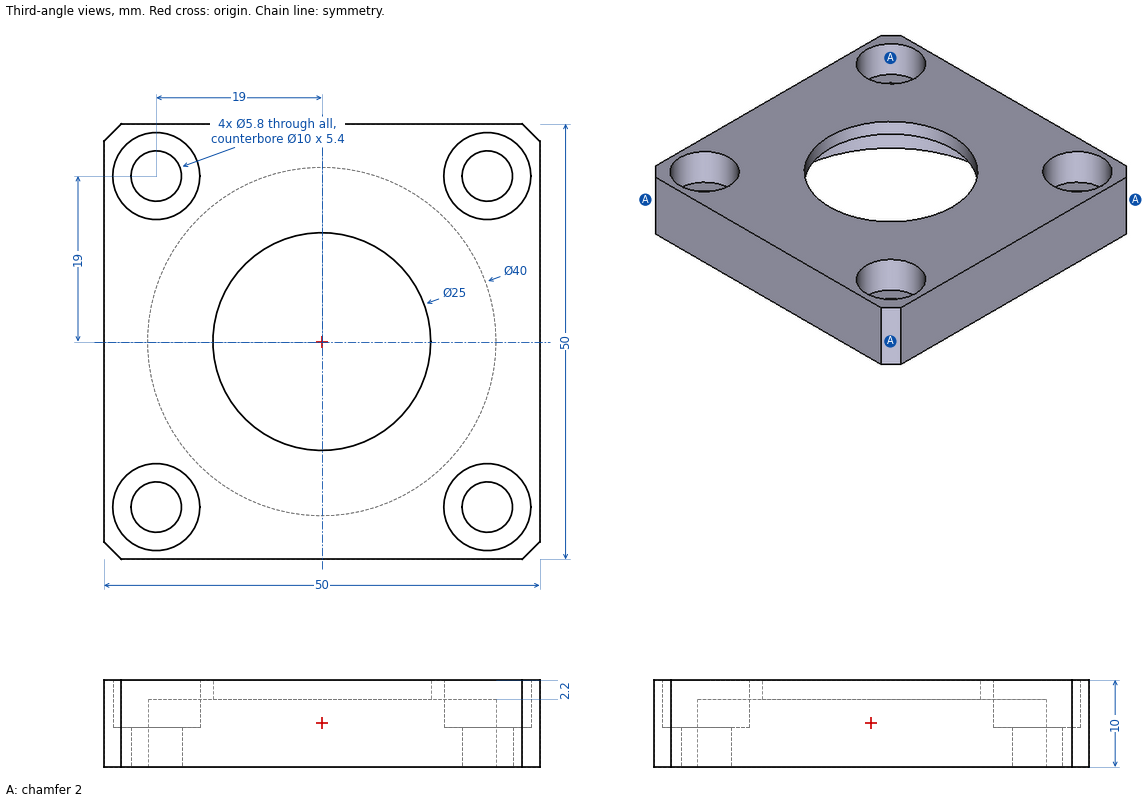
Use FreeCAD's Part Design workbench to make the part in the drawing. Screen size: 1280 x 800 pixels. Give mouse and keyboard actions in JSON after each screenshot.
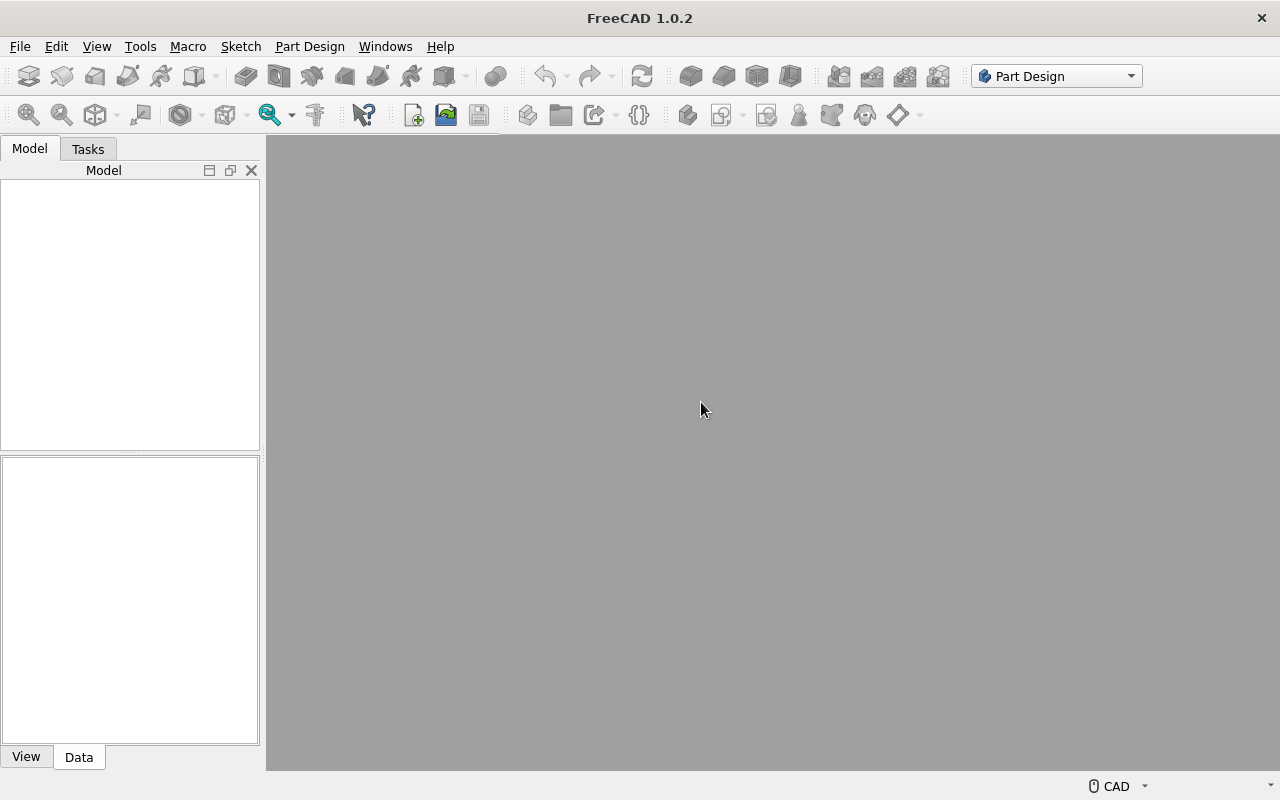
{"action": "left_click", "coordinate": [413, 116]}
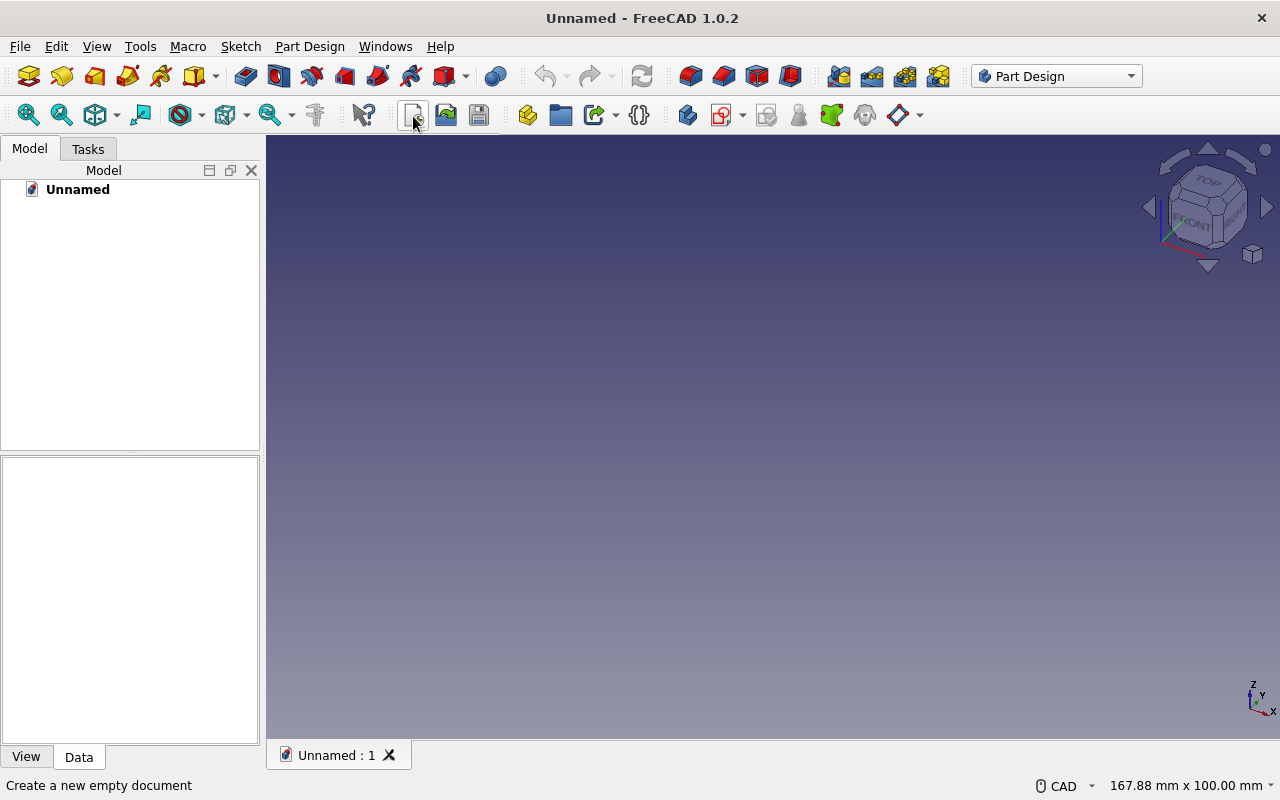
{"action": "left_click", "coordinate": [720, 116]}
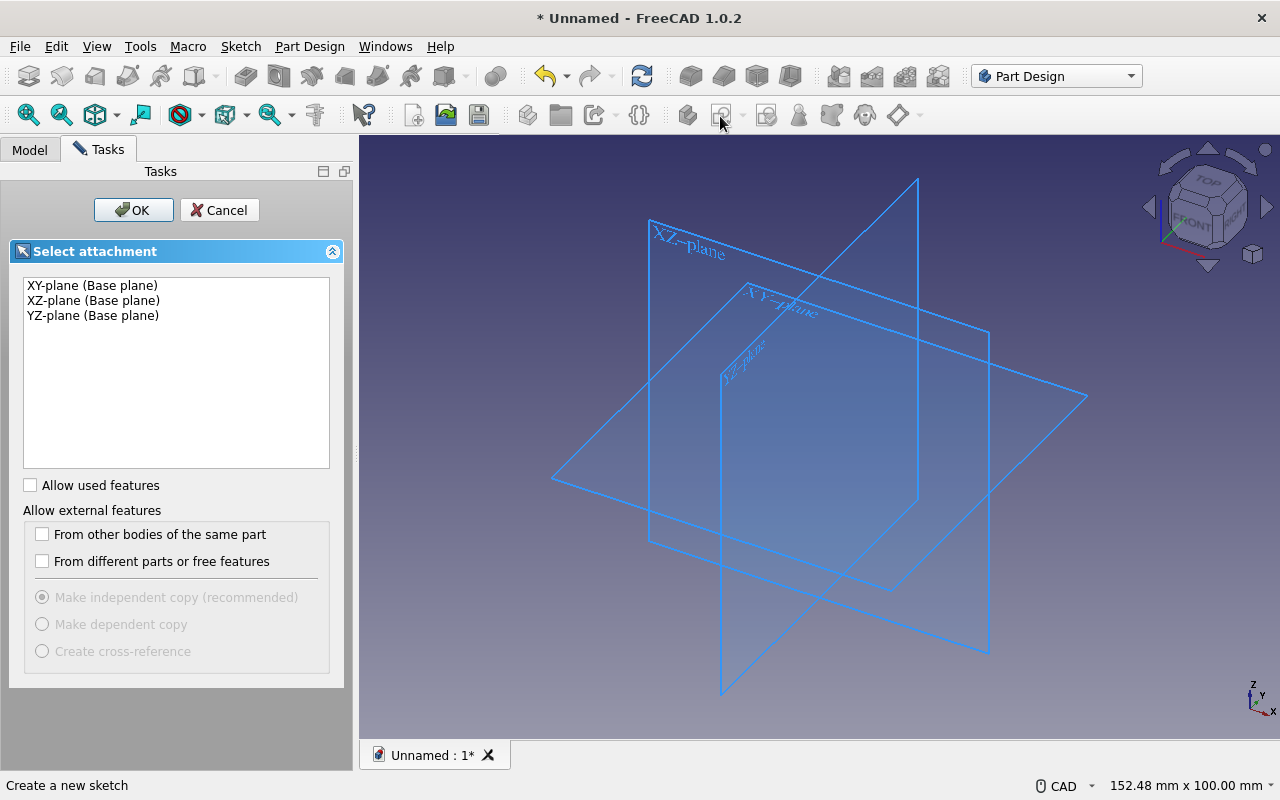
{"action": "left_click", "coordinate": [84, 286]}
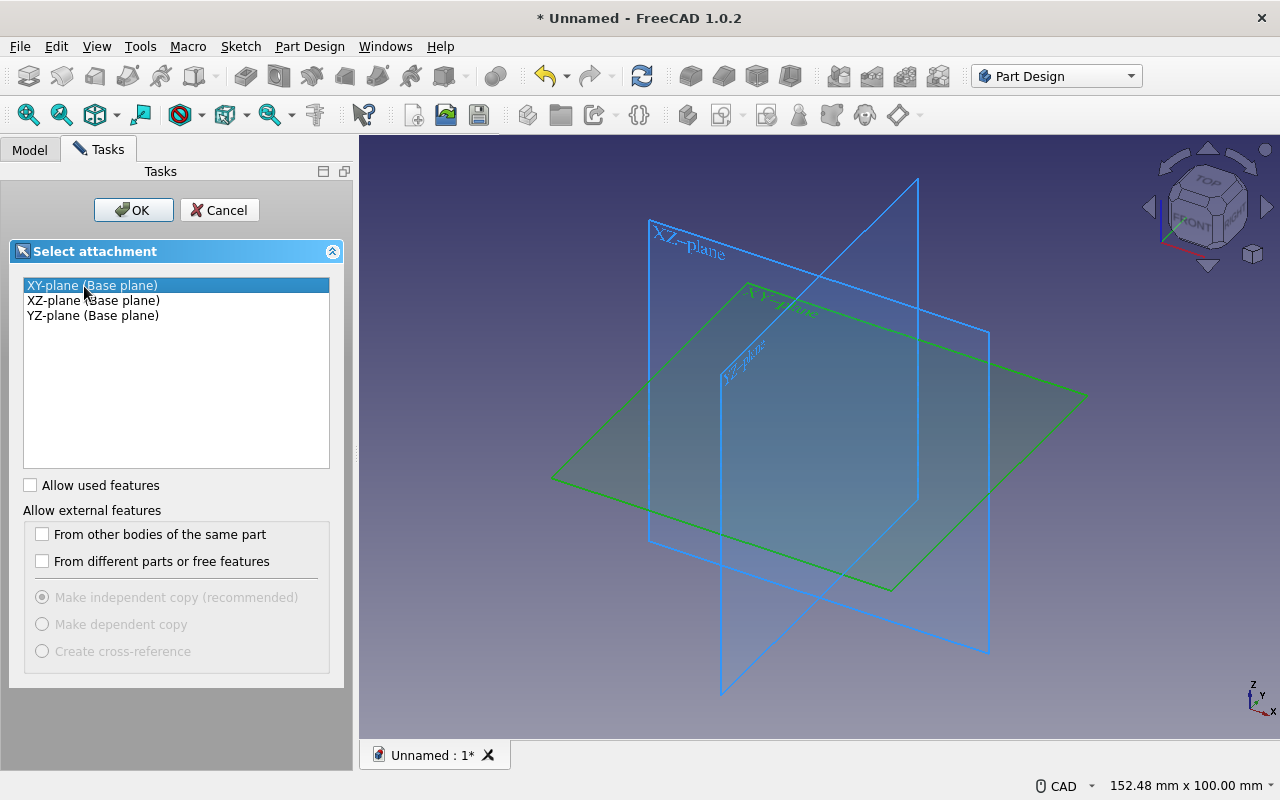
{"action": "left_click", "coordinate": [134, 210]}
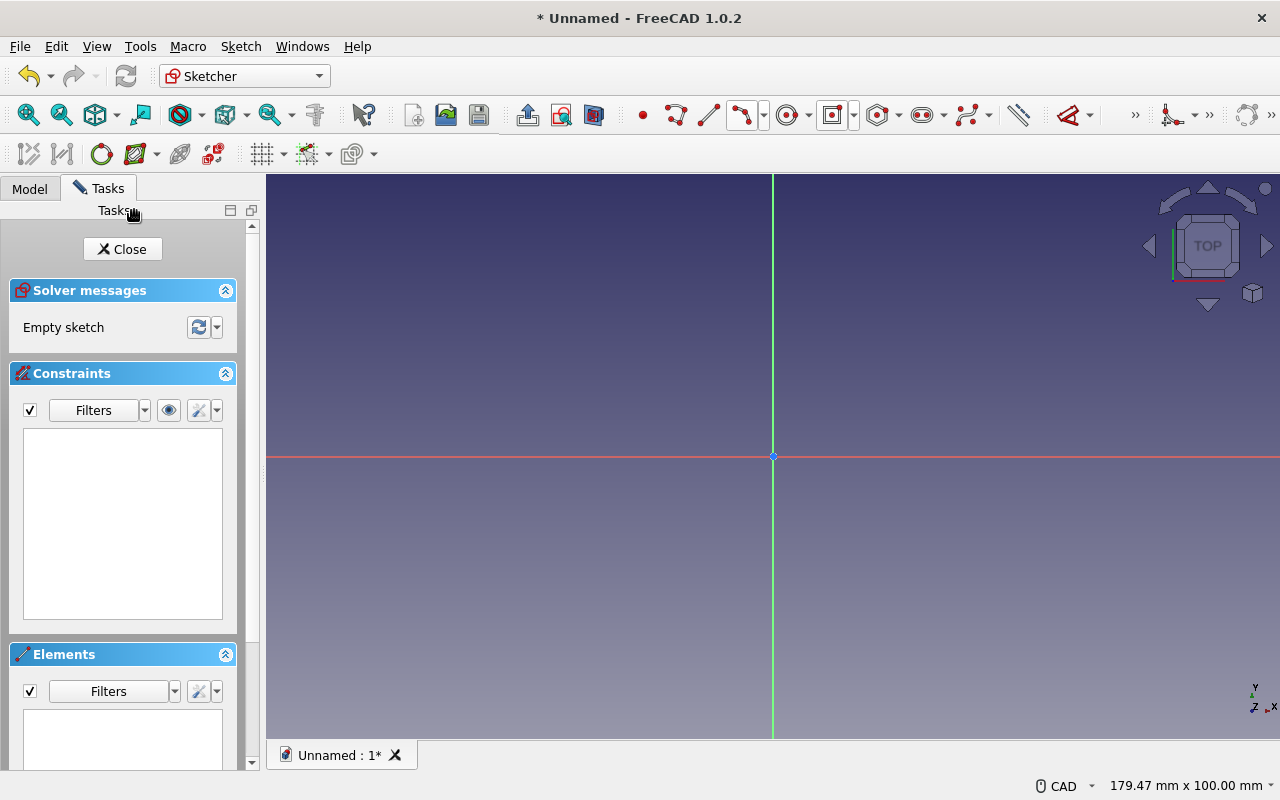
{"action": "left_click", "coordinate": [832, 116]}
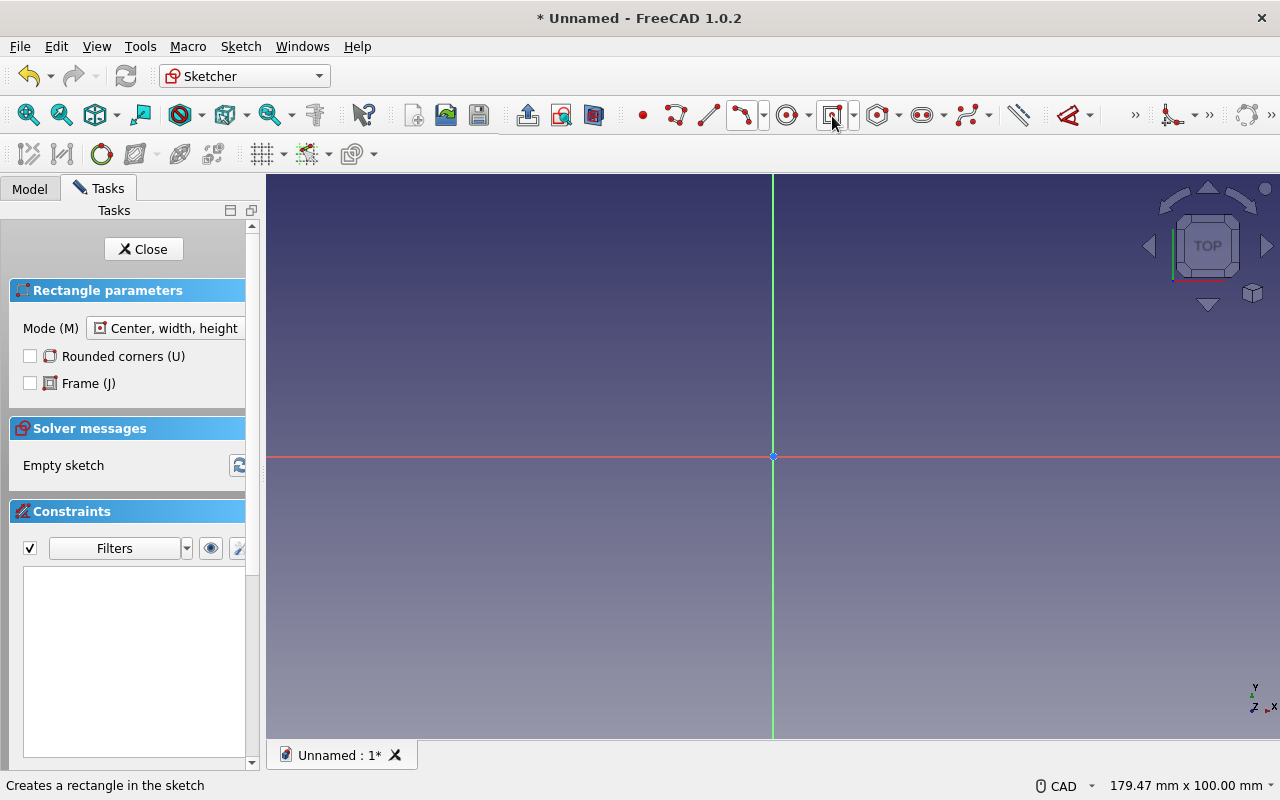
{"action": "left_click", "coordinate": [773, 456]}
{"action": "mouse_move", "coordinate": [914, 315]}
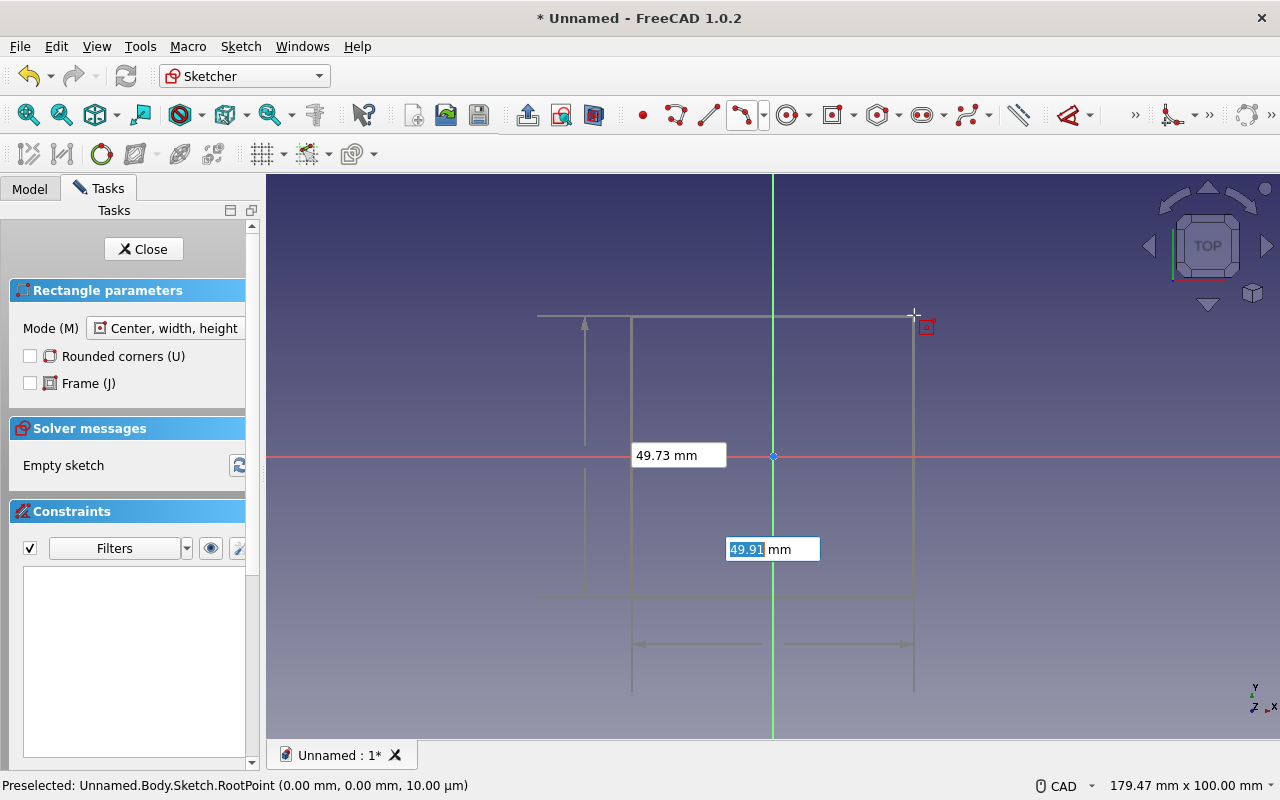
{"action": "type", "text": "50"}
{"action": "key", "text": "Tab"}
{"action": "type", "text": "50"}
{"action": "key", "text": "Return"}
{"action": "key", "text": "Escape"}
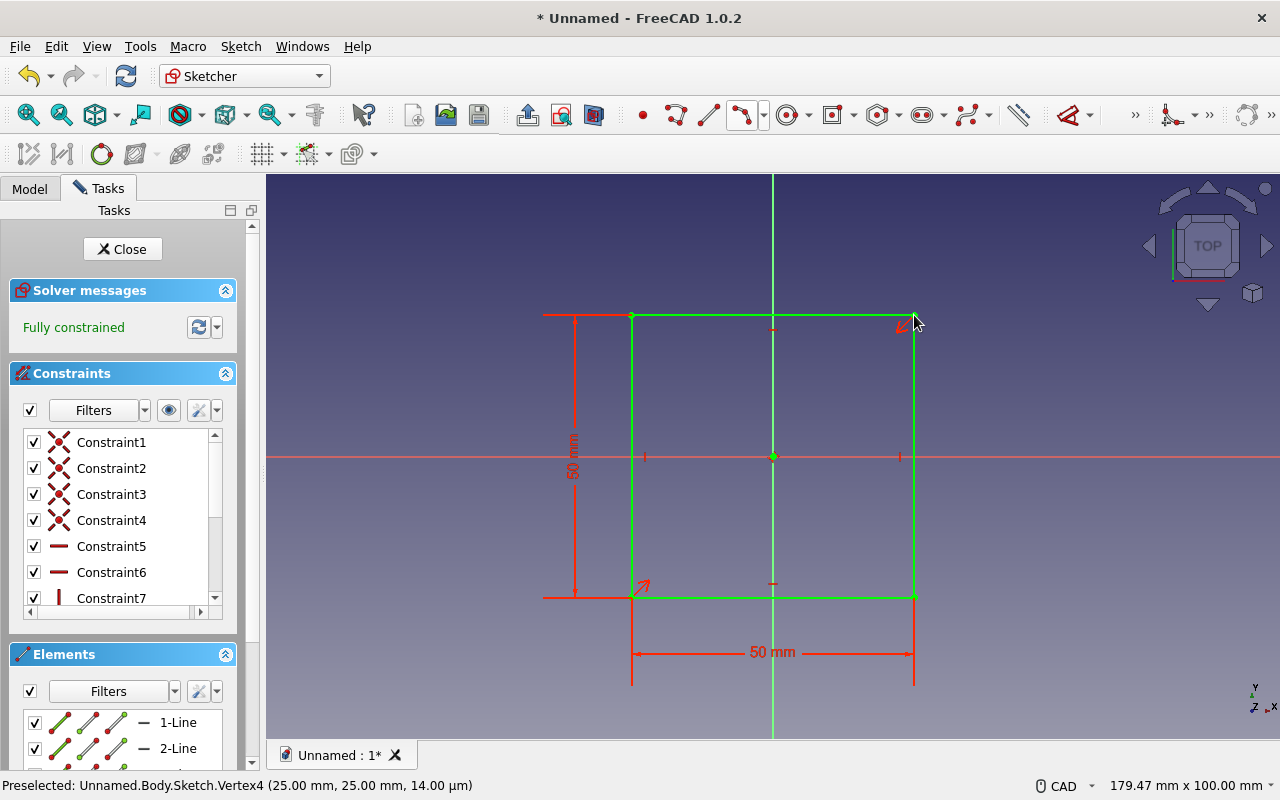
{"action": "left_click", "coordinate": [123, 249]}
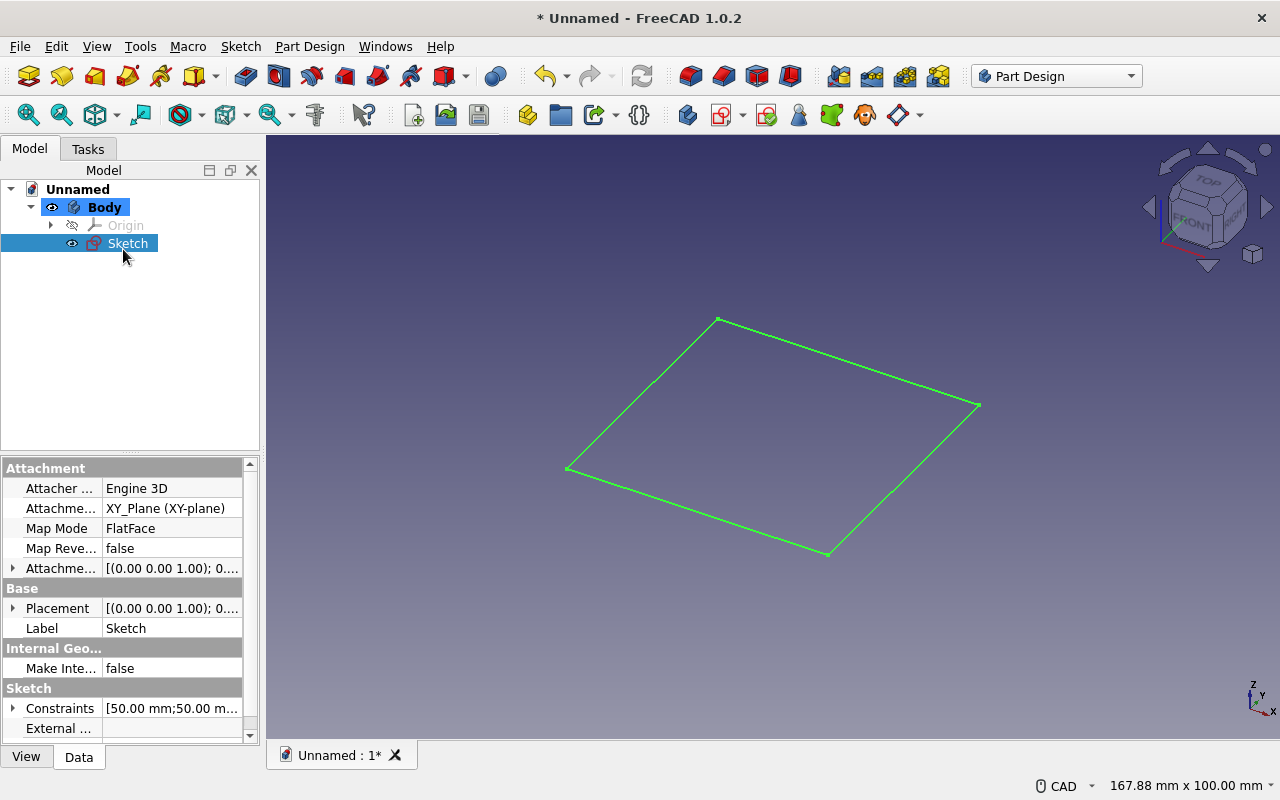
{"action": "left_click", "coordinate": [29, 76]}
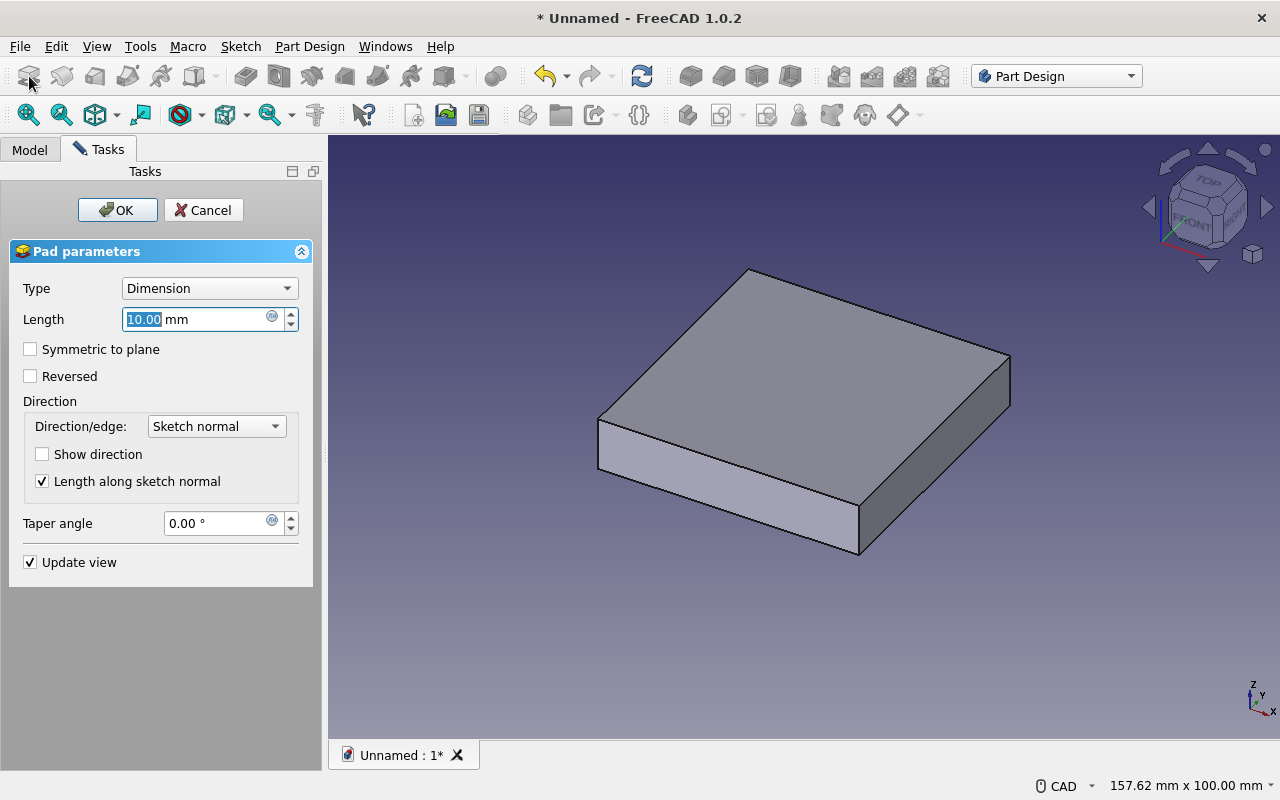
{"action": "type", "text": "10"}
{"action": "key", "text": "Tab"}